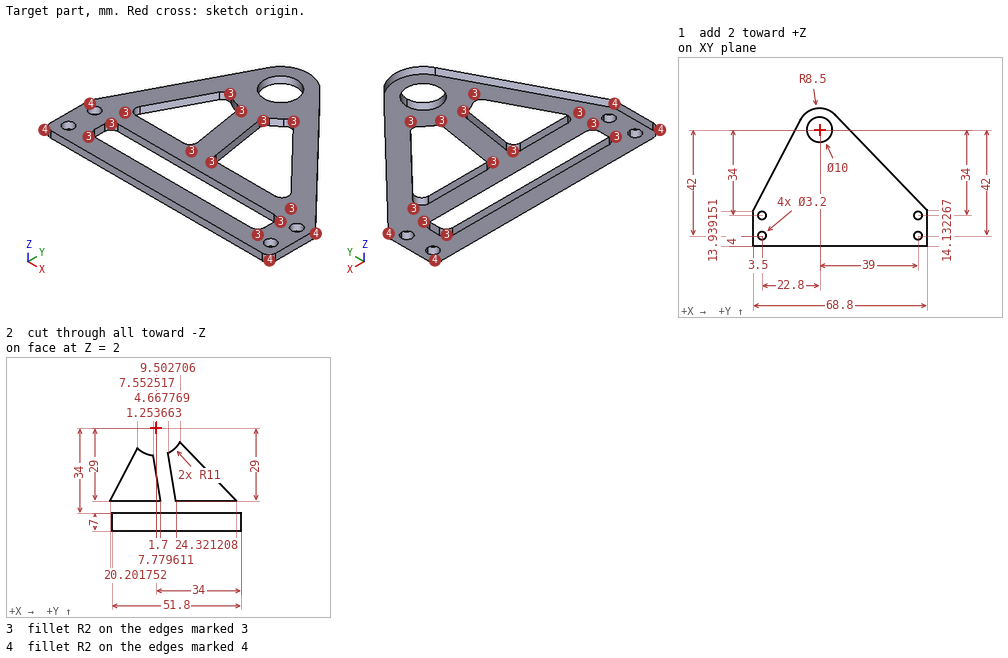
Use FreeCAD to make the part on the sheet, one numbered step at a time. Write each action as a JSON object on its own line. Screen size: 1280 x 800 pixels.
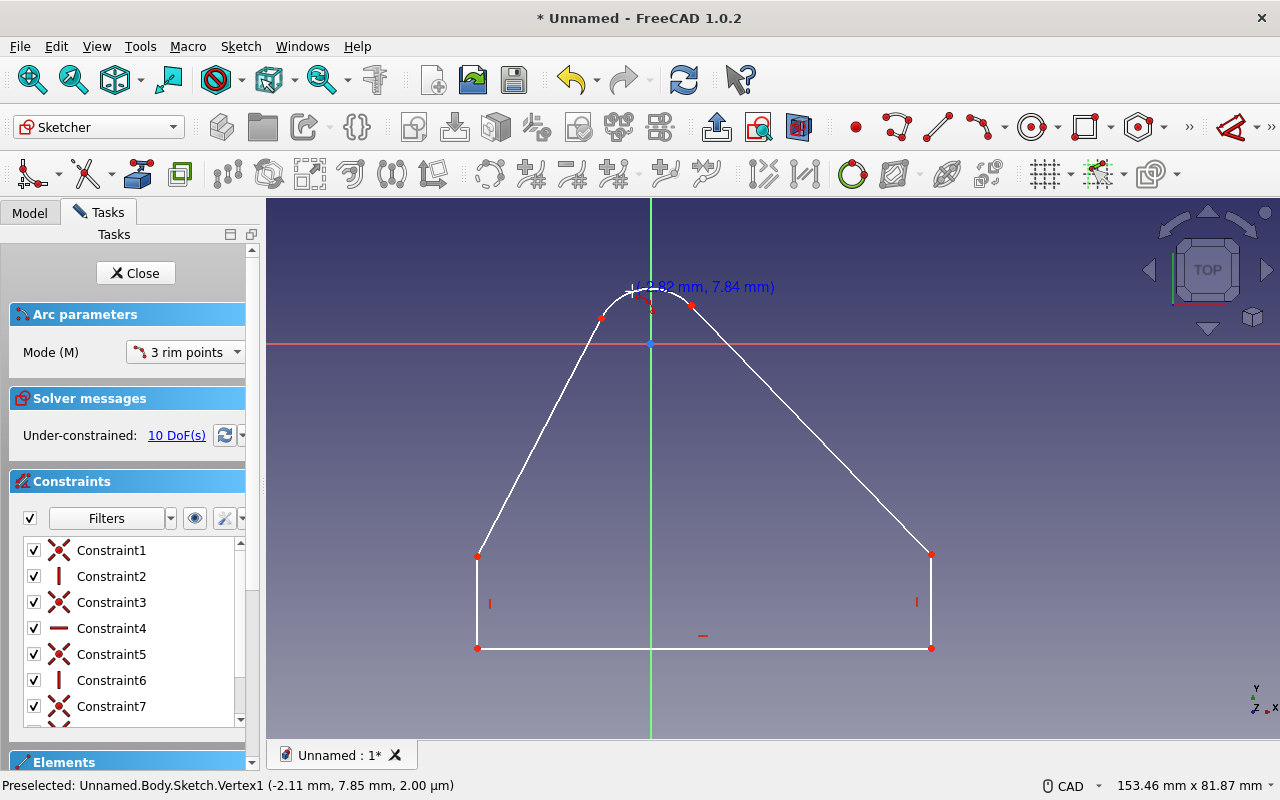
{"action": "key", "text": "g c"}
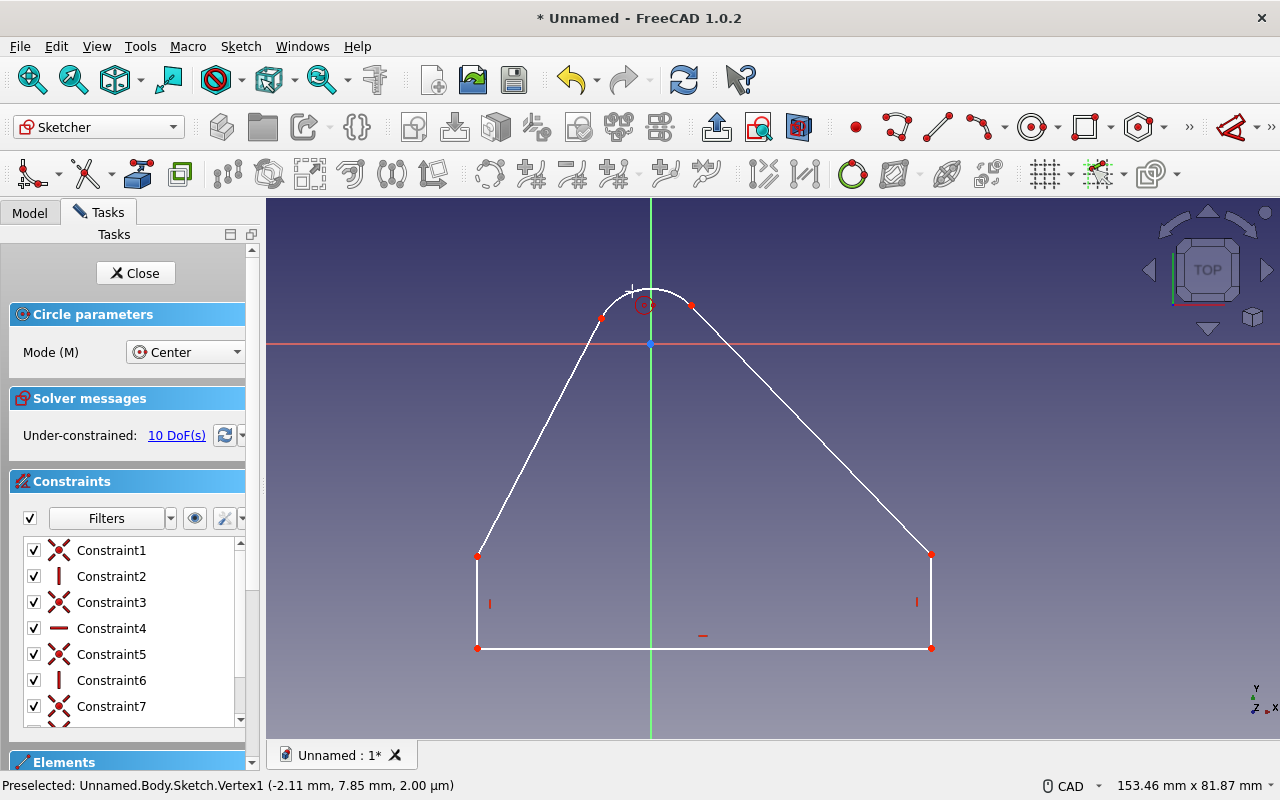
{"action": "scroll", "coordinate": [500, 621], "scroll_direction": "up", "scroll_amount": 4}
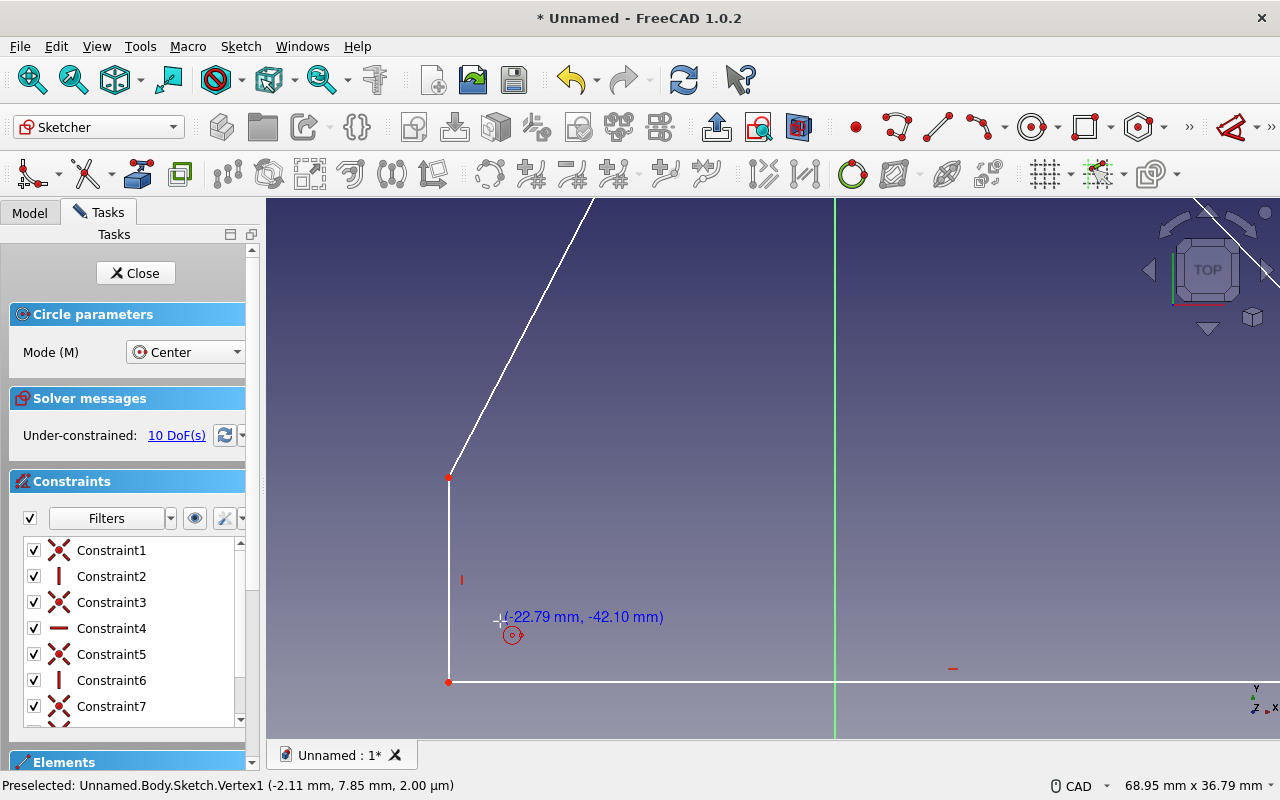
{"action": "left_click", "coordinate": [500, 621]}
{"action": "left_click", "coordinate": [516, 604]}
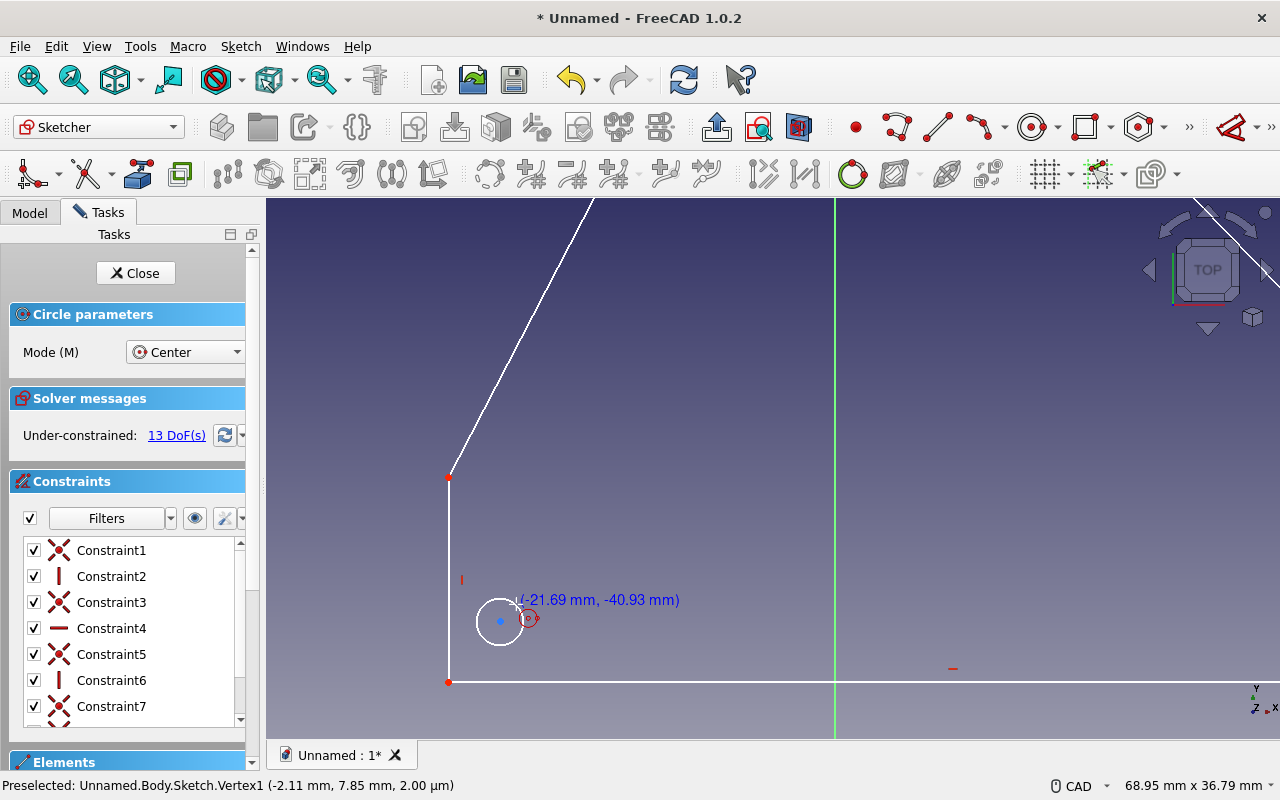
{"action": "left_click", "coordinate": [500, 503]}
{"action": "left_click", "coordinate": [516, 487]}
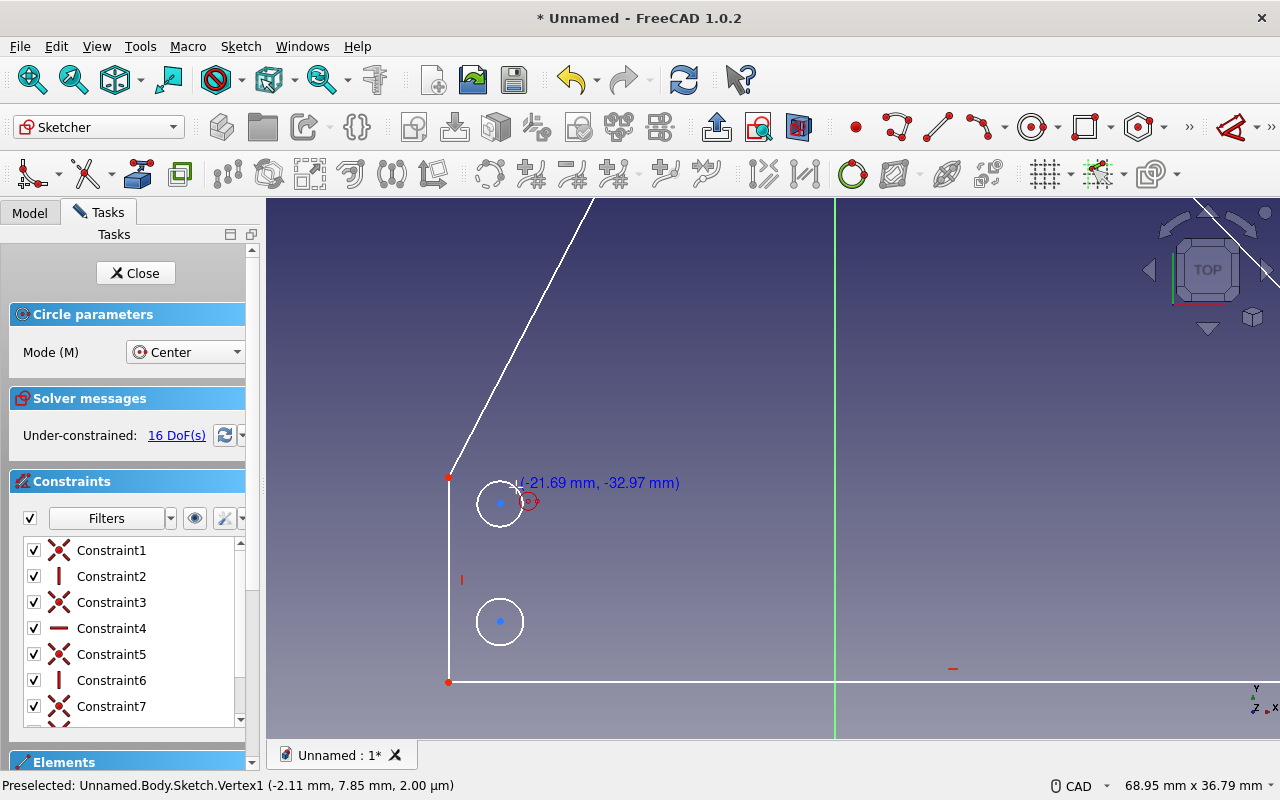
{"action": "scroll", "coordinate": [501, 623], "scroll_direction": "down", "scroll_amount": 4}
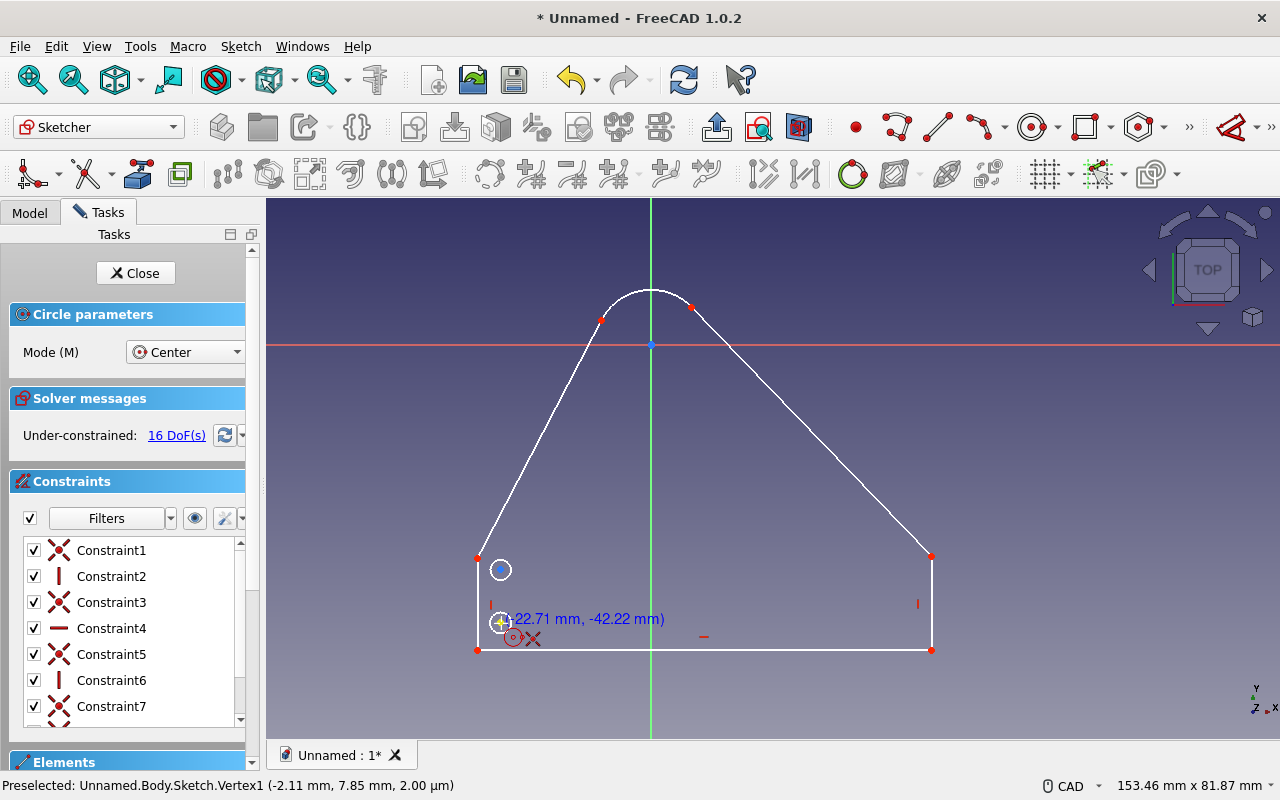
{"action": "scroll", "coordinate": [909, 622], "scroll_direction": "up", "scroll_amount": 4}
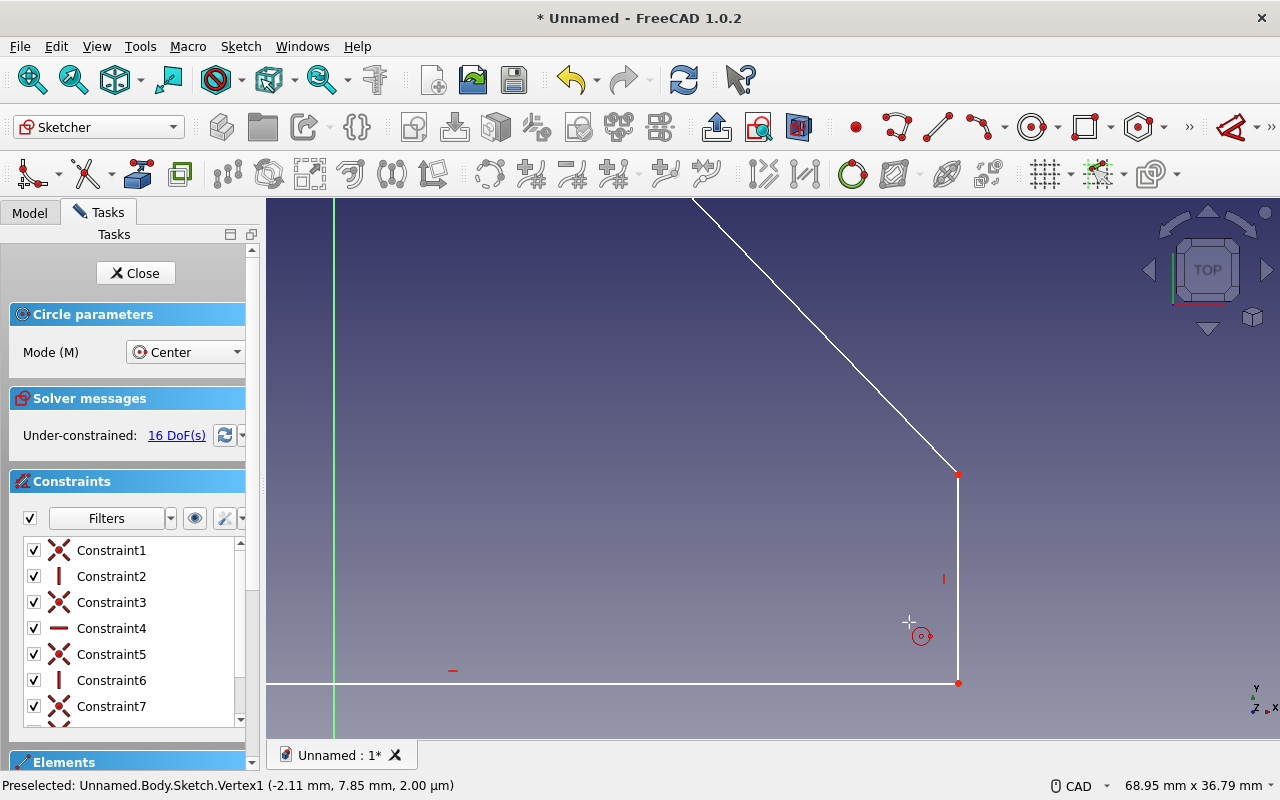
{"action": "left_click", "coordinate": [908, 622]}
{"action": "left_click", "coordinate": [925, 605]}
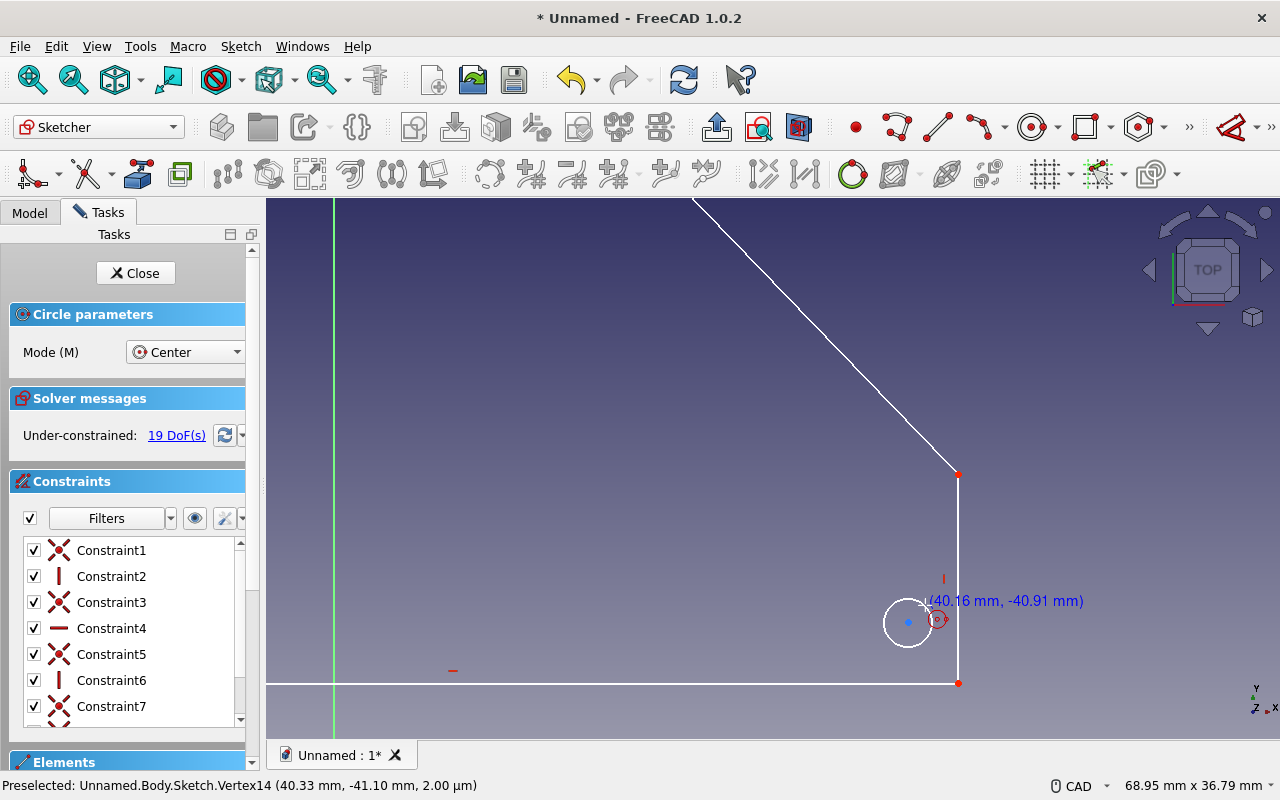
{"action": "left_click", "coordinate": [908, 504]}
{"action": "left_click", "coordinate": [925, 488]}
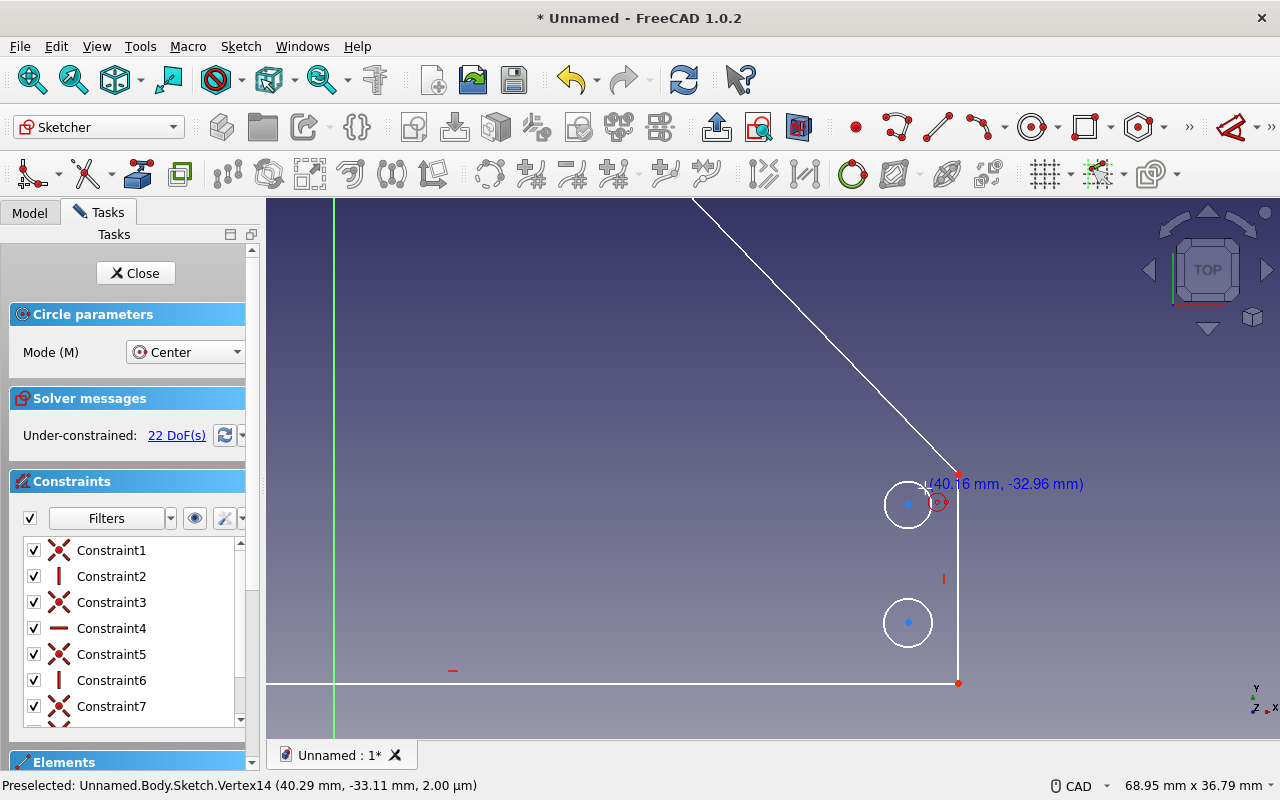
{"action": "scroll", "coordinate": [909, 622], "scroll_direction": "down", "scroll_amount": 4}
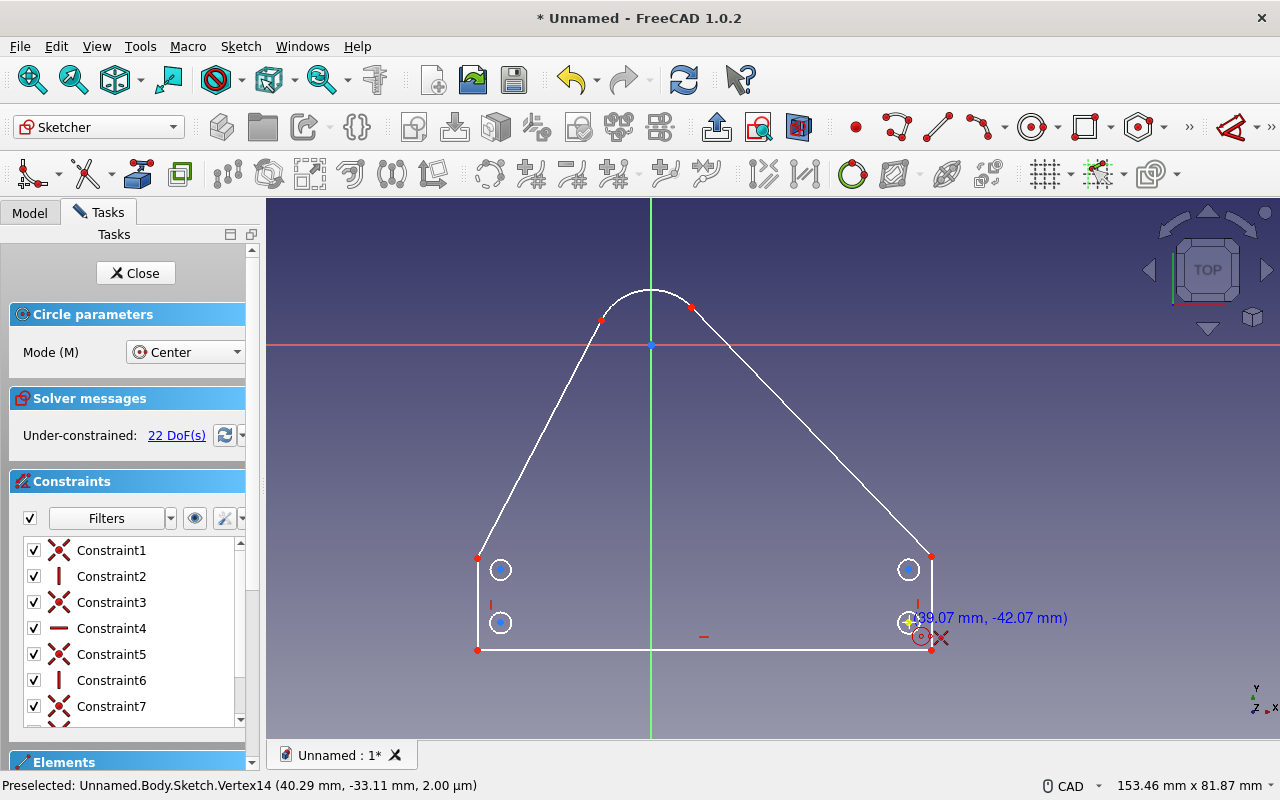
{"action": "left_click", "coordinate": [651, 345]}
{"action": "left_click", "coordinate": [675, 322]}
{"action": "key", "text": "Escape"}